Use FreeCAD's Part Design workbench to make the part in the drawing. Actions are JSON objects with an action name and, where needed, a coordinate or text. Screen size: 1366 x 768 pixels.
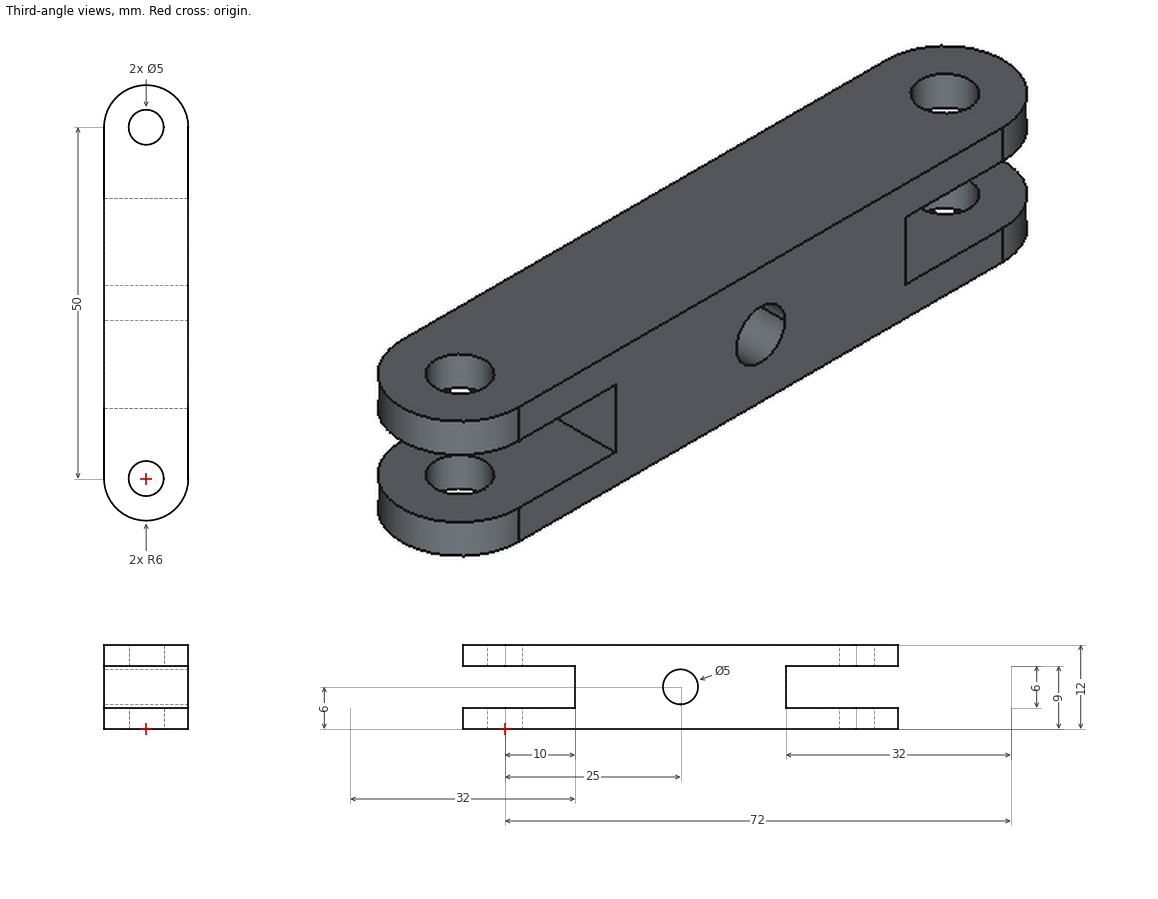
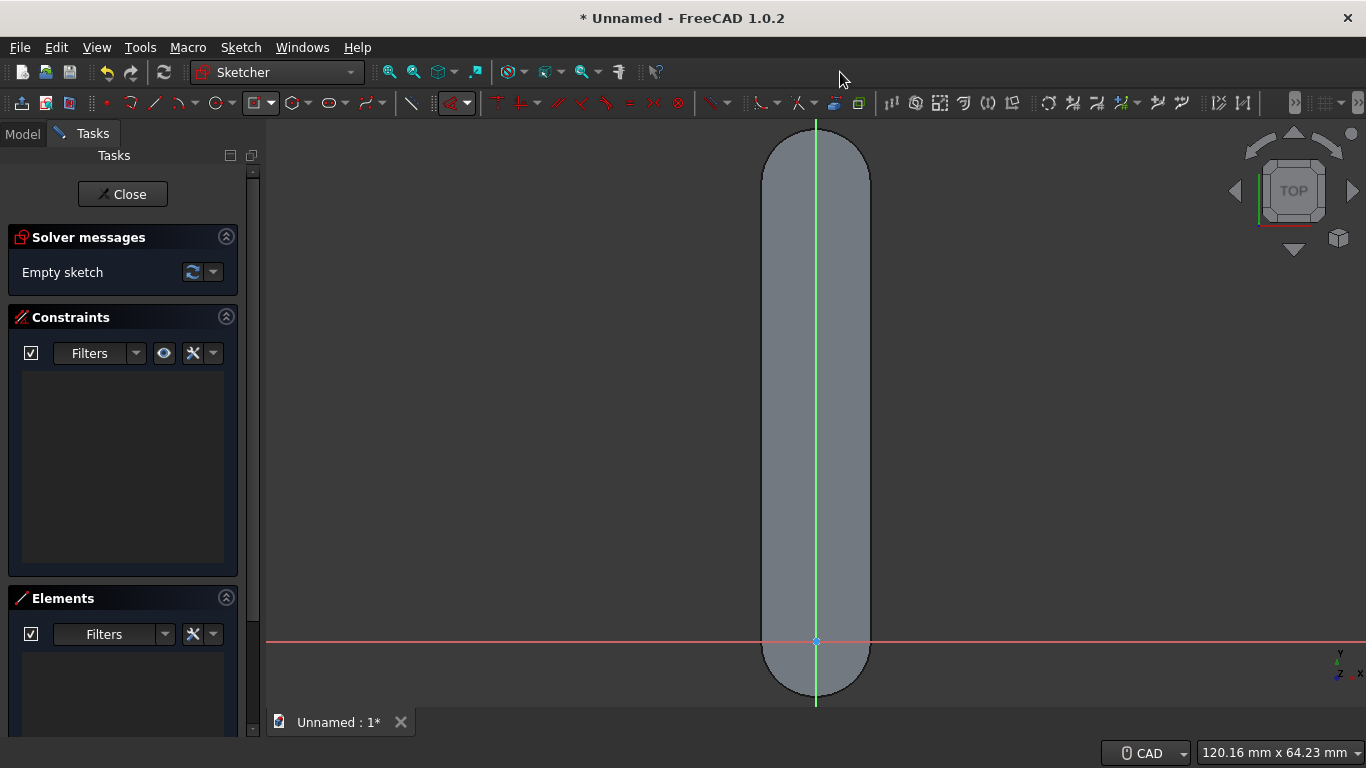
{"action": "scroll", "coordinate": [438, 413], "scroll_direction": "down", "scroll_amount": 1}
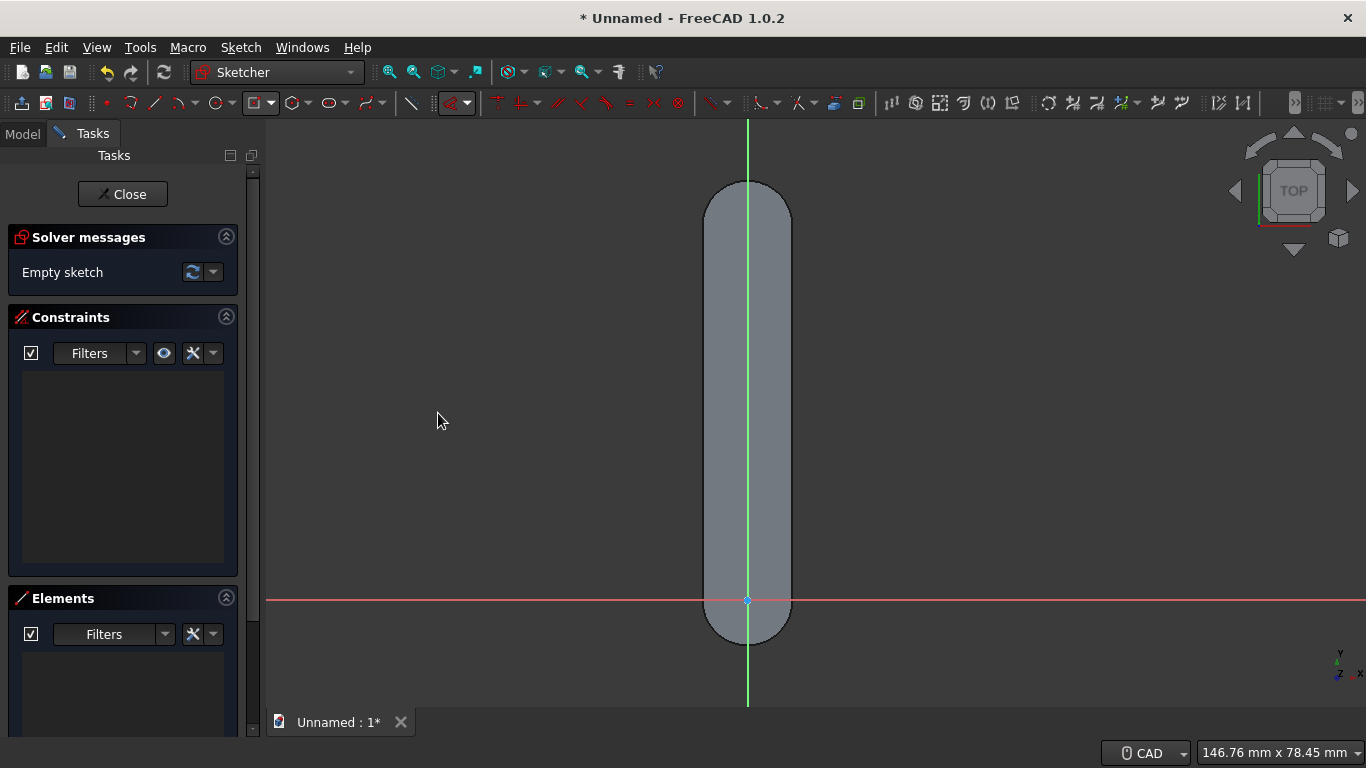
{"action": "key", "text": "g c"}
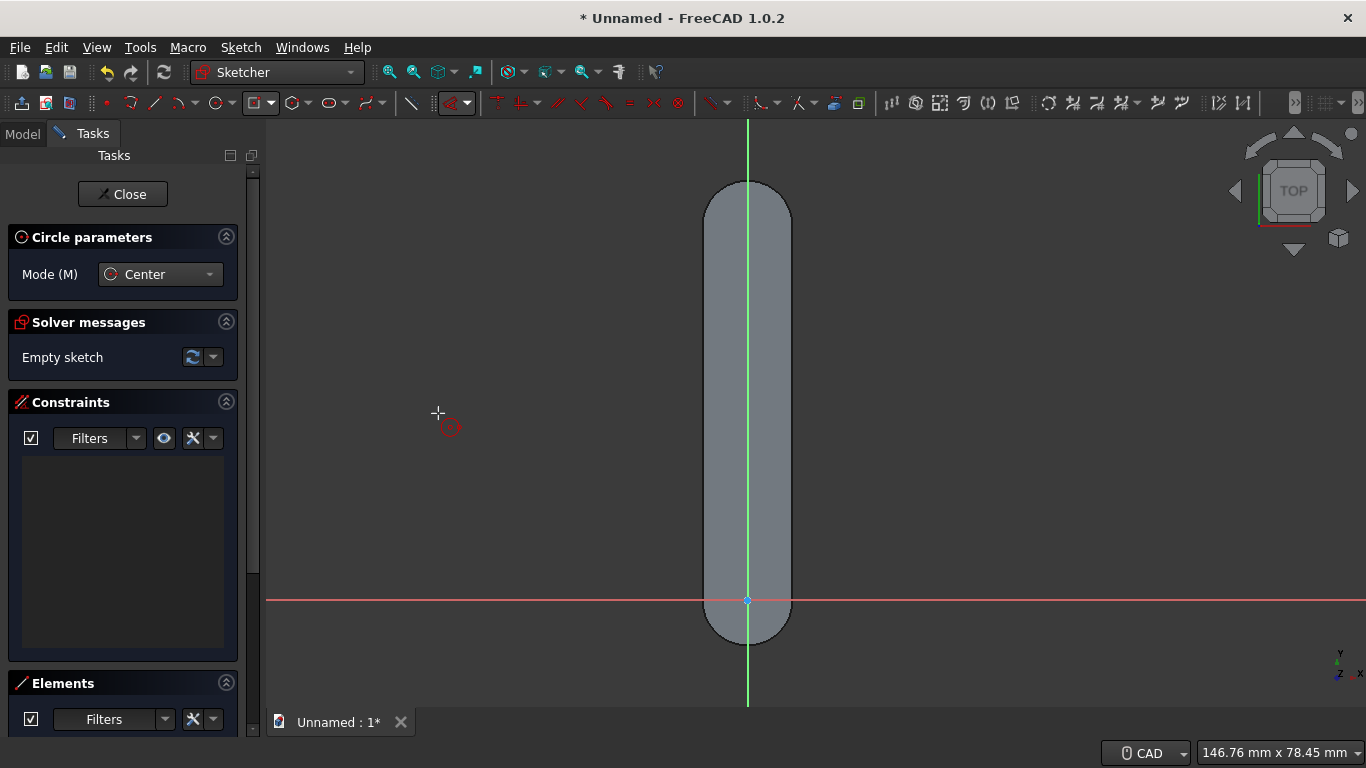
{"action": "left_click", "coordinate": [748, 226]}
{"action": "left_click", "coordinate": [765, 219]}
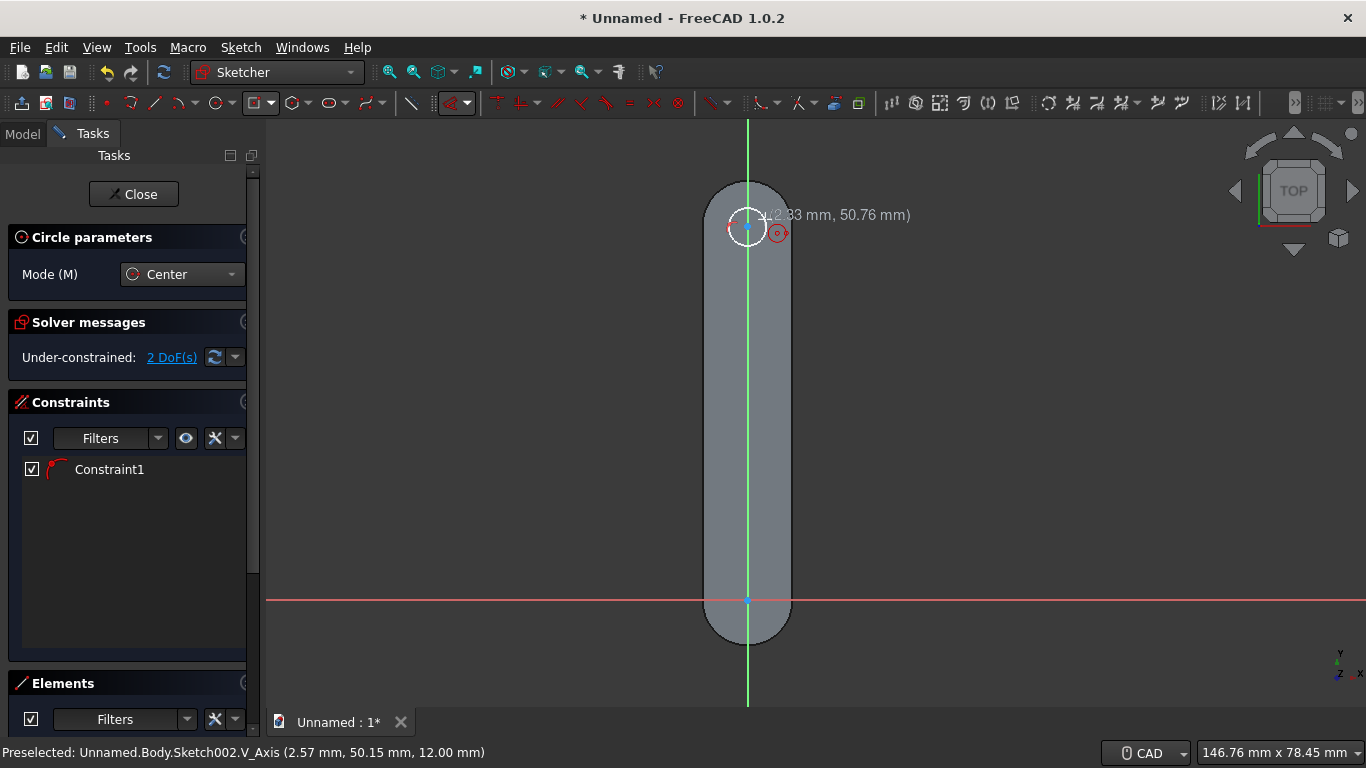
{"action": "left_click", "coordinate": [748, 600]}
{"action": "left_click", "coordinate": [761, 587]}
{"action": "key", "text": "Escape"}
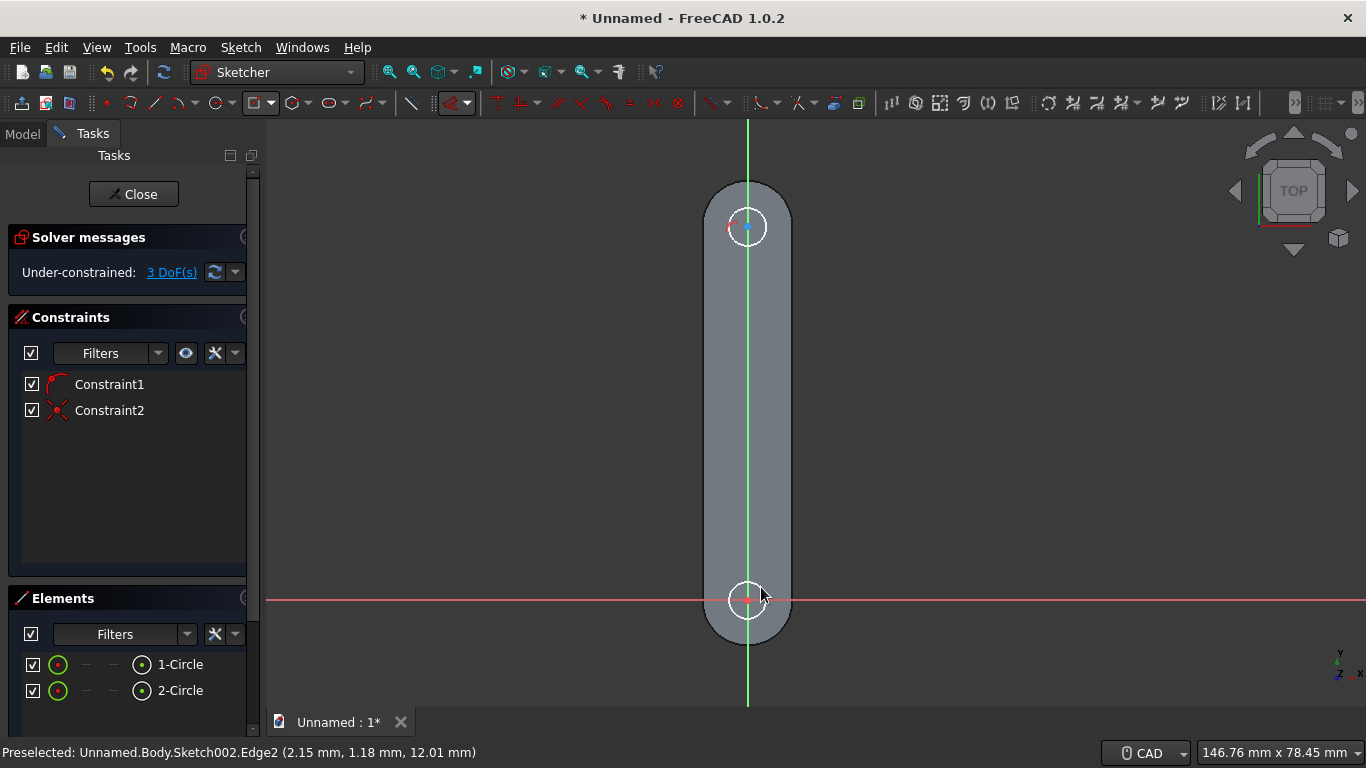
{"action": "left_click", "coordinate": [761, 214]}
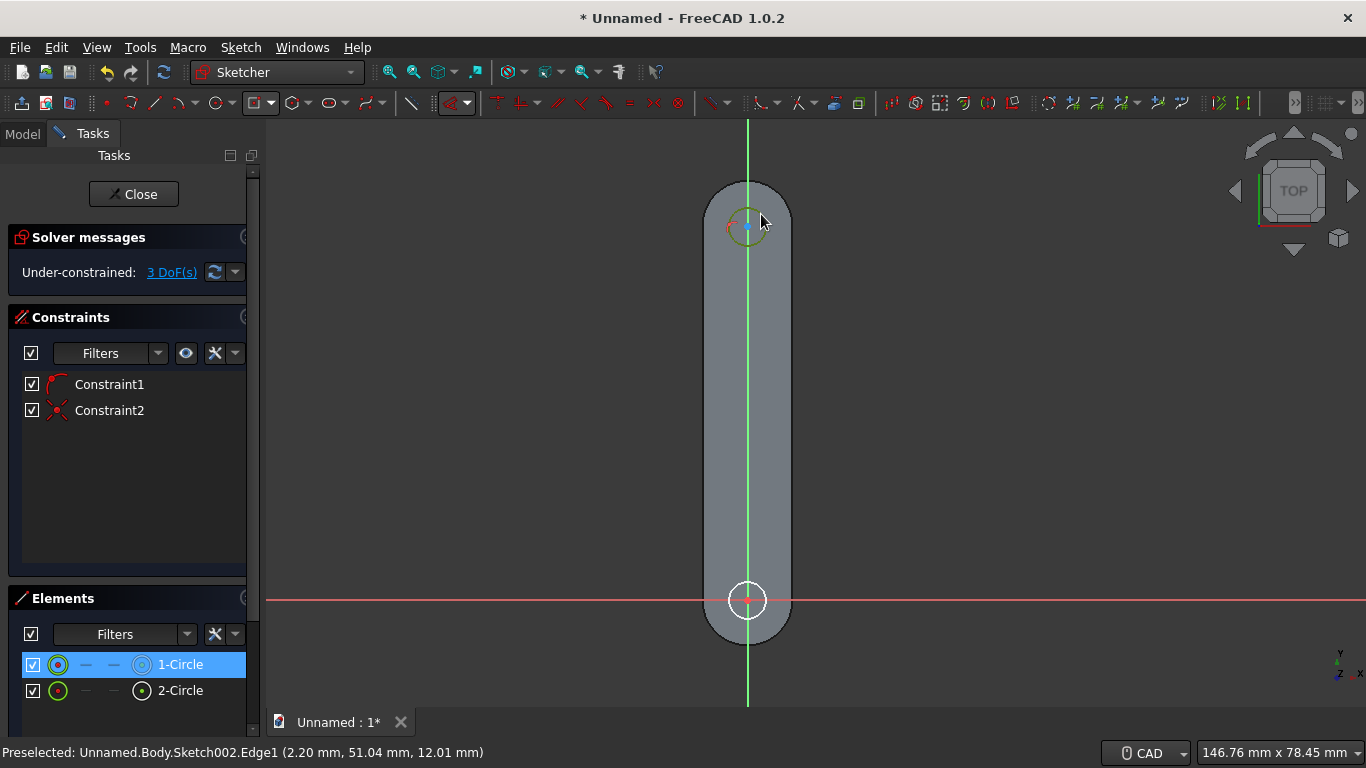
{"action": "left_click", "coordinate": [760, 587]}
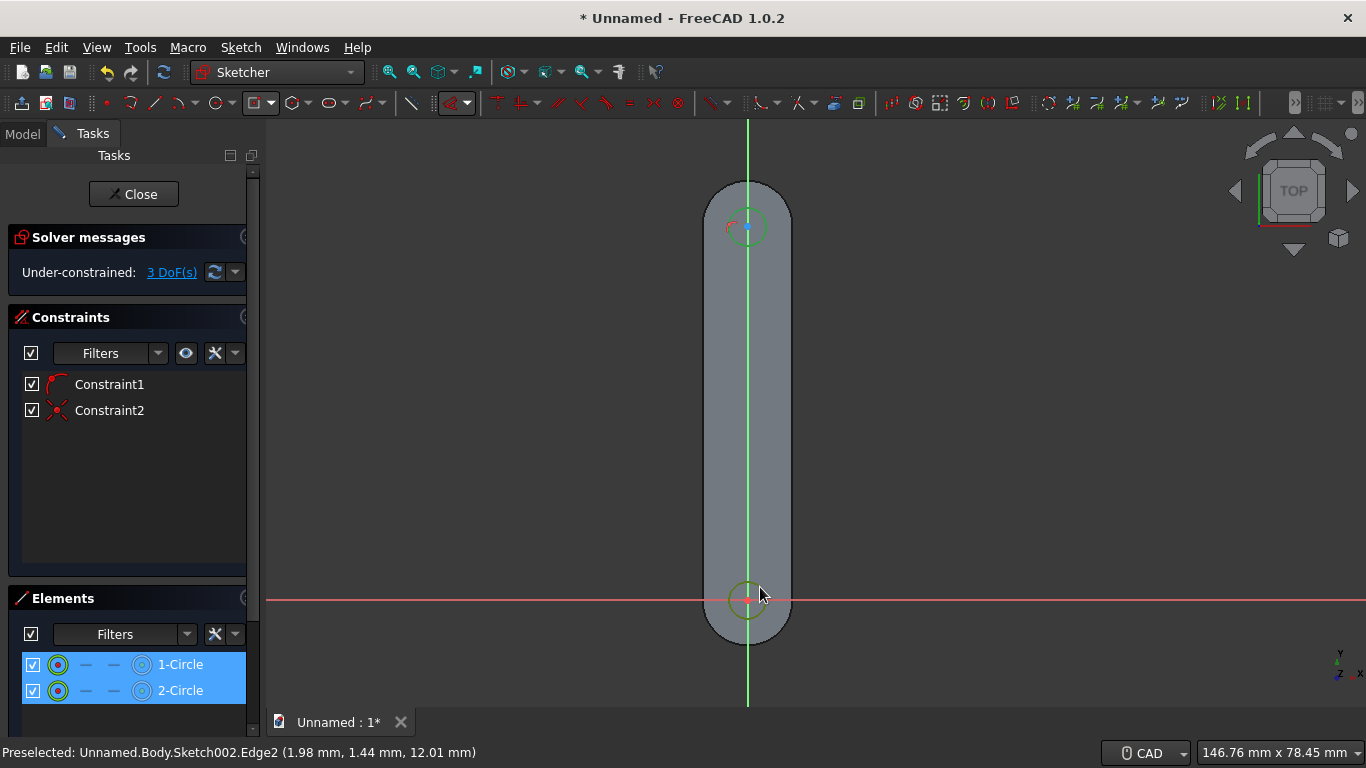
{"action": "key", "text": "e"}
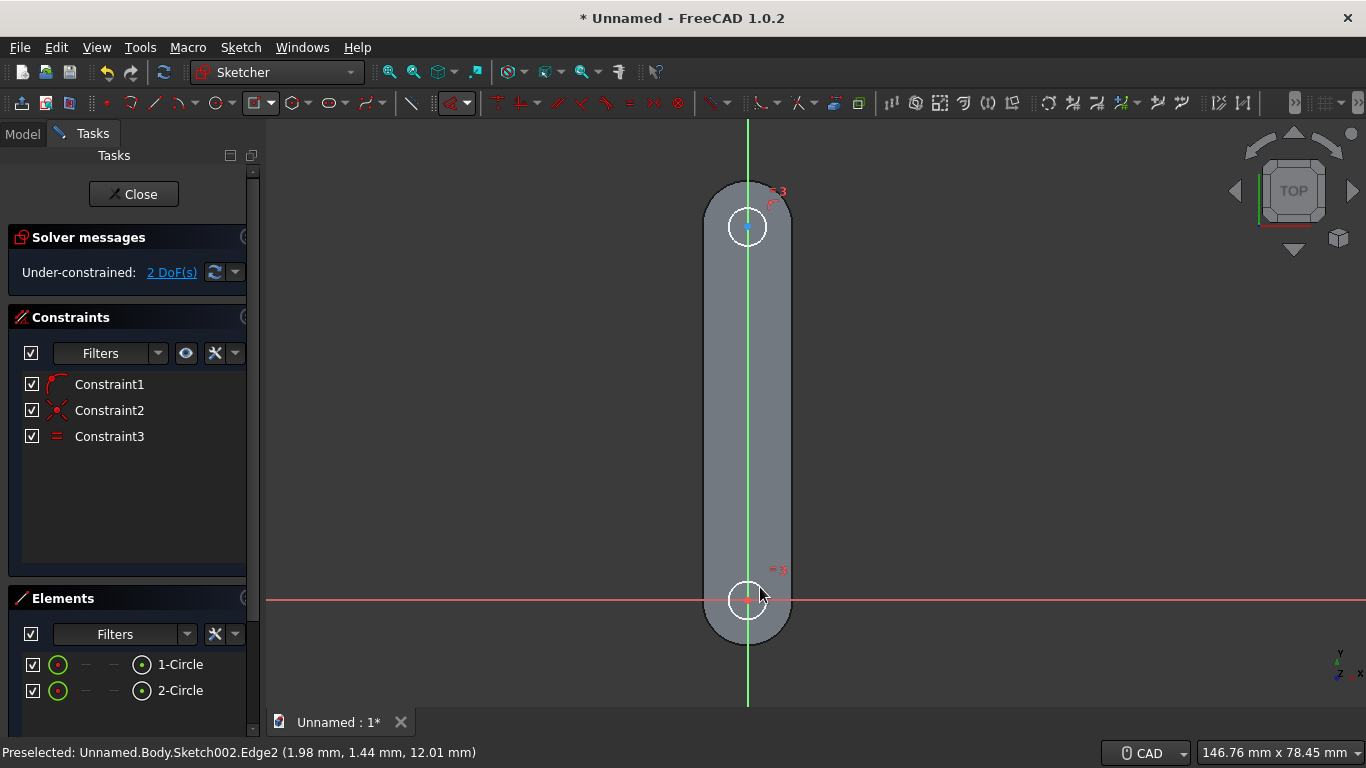
{"action": "left_click", "coordinate": [761, 214]}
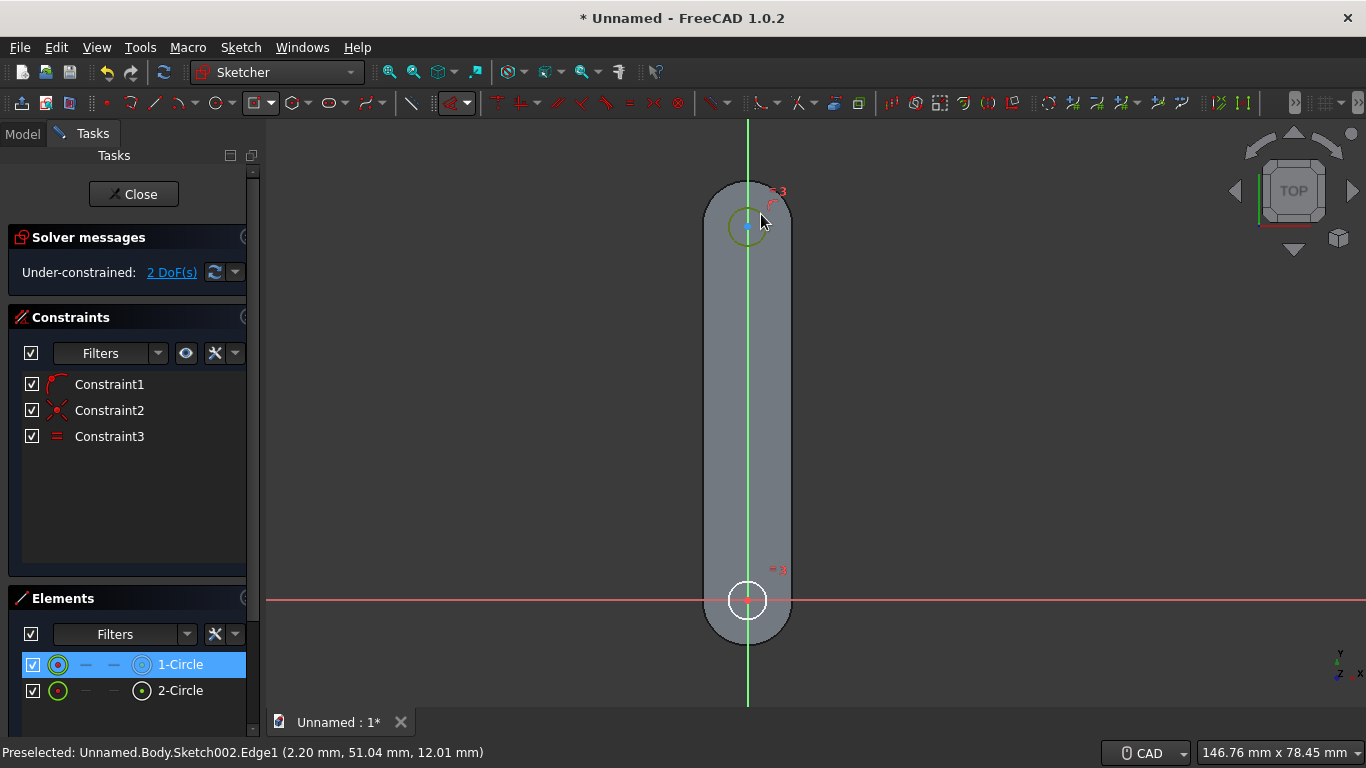
{"action": "key", "text": "k o"}